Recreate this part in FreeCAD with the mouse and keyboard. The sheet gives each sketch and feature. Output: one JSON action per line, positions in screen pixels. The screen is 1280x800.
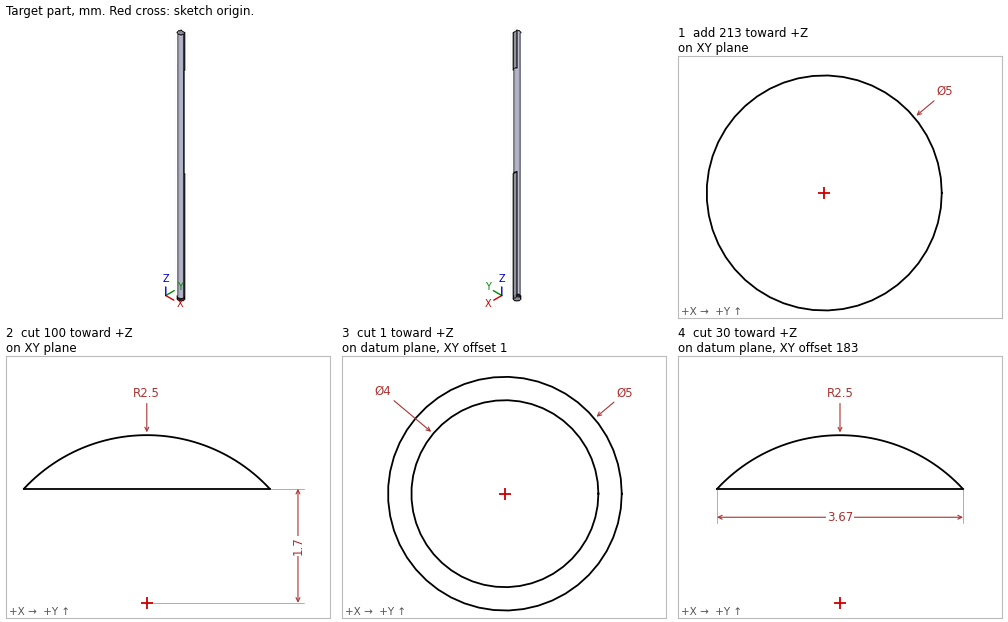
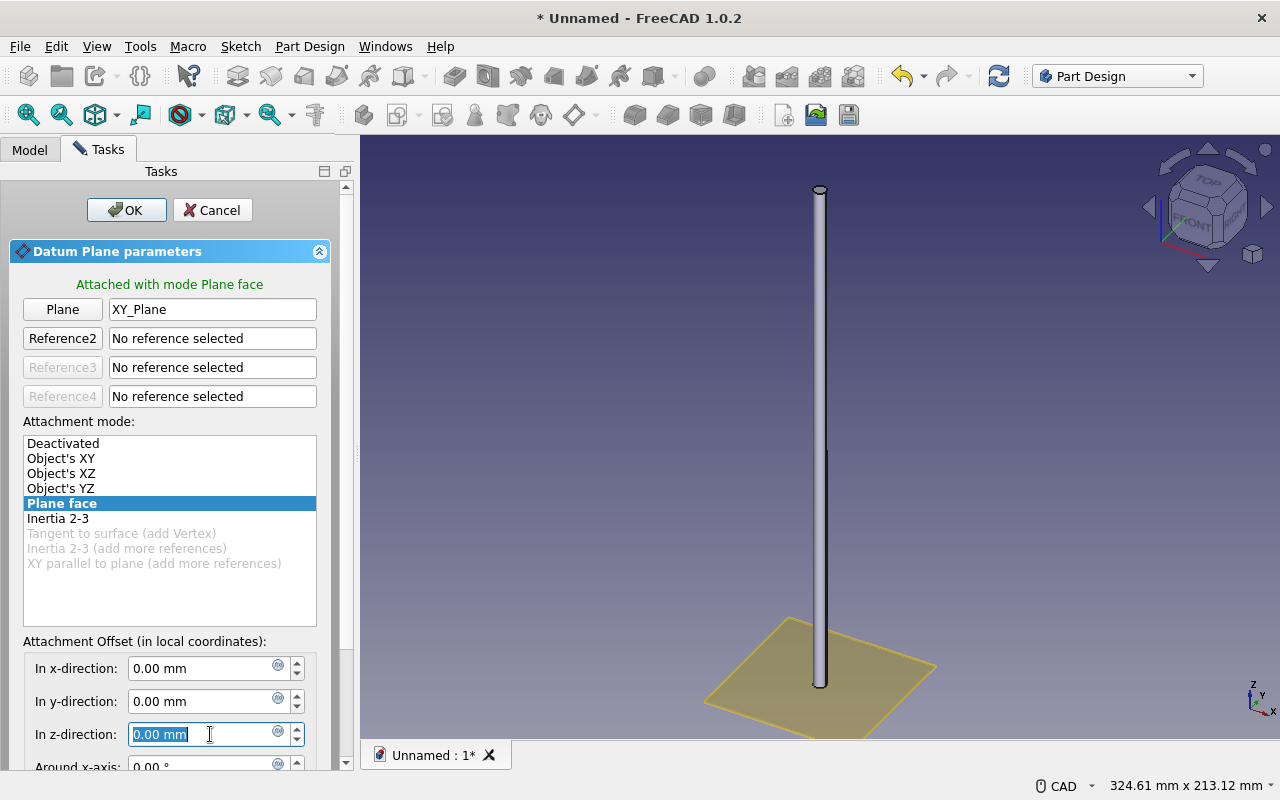
{"action": "type", "text": "1"}
{"action": "key", "text": "Tab"}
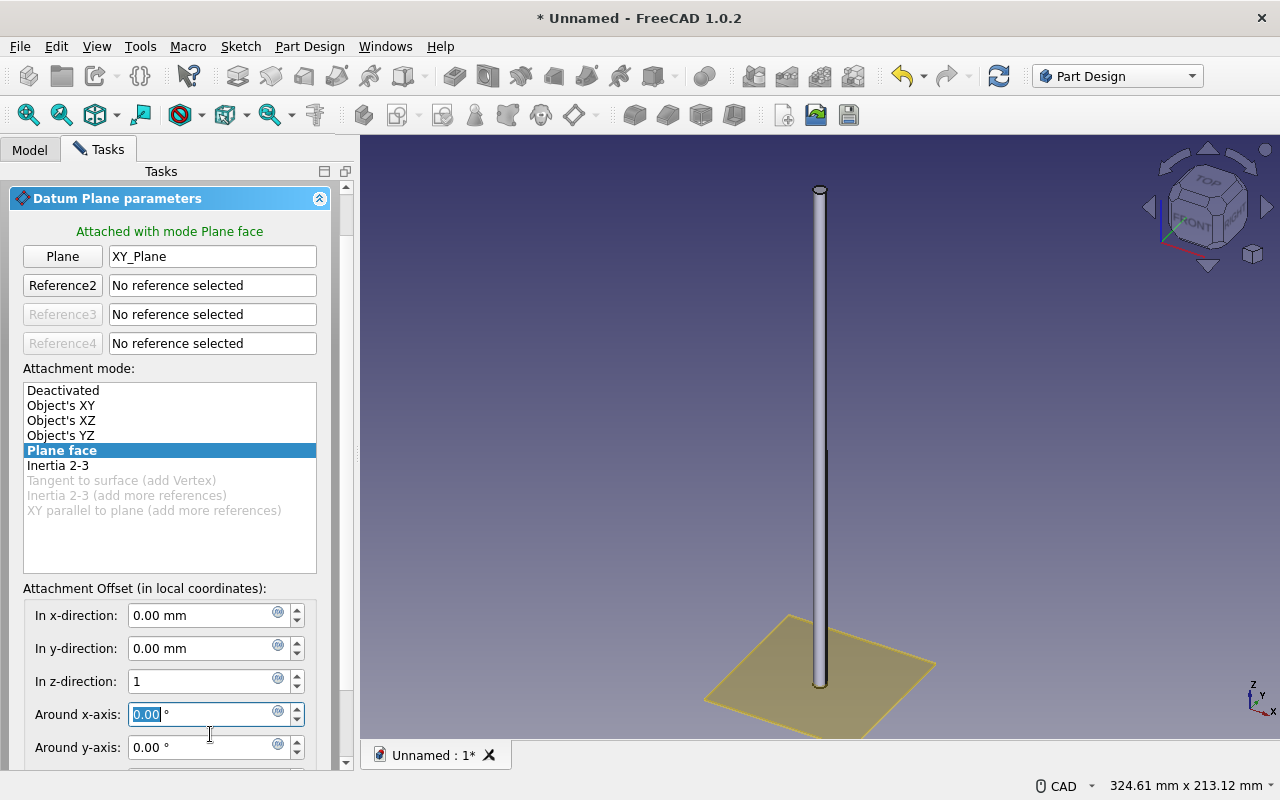
{"action": "scroll", "coordinate": [346, 476], "scroll_direction": "up", "scroll_amount": 2}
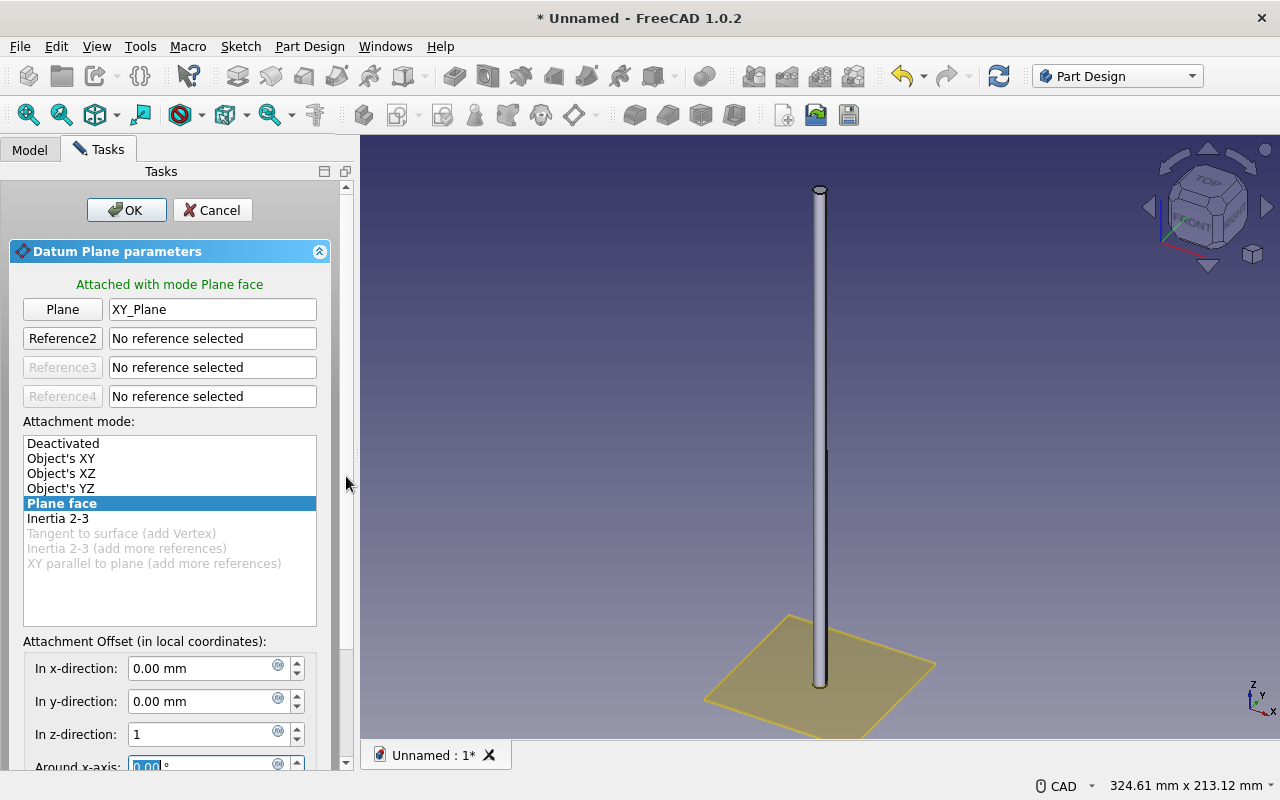
{"action": "left_click", "coordinate": [127, 210]}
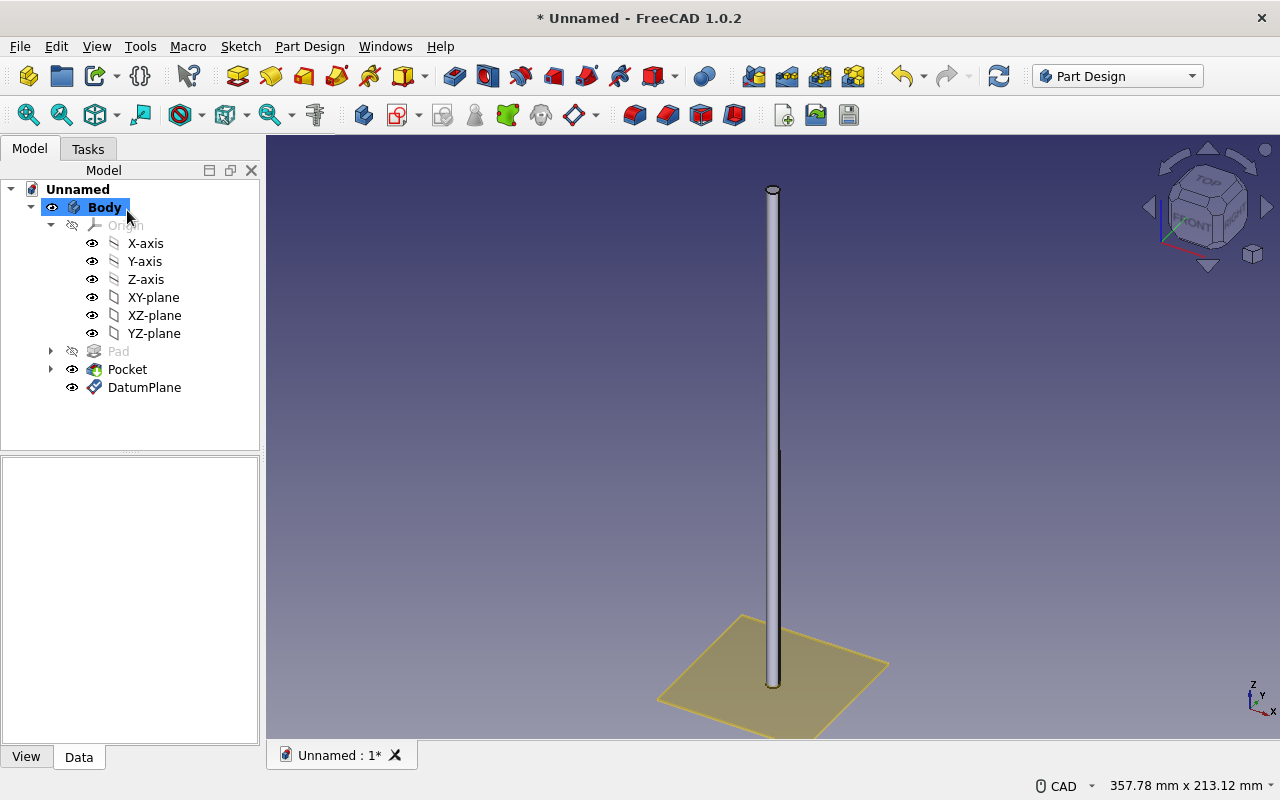
{"action": "left_click", "coordinate": [117, 387]}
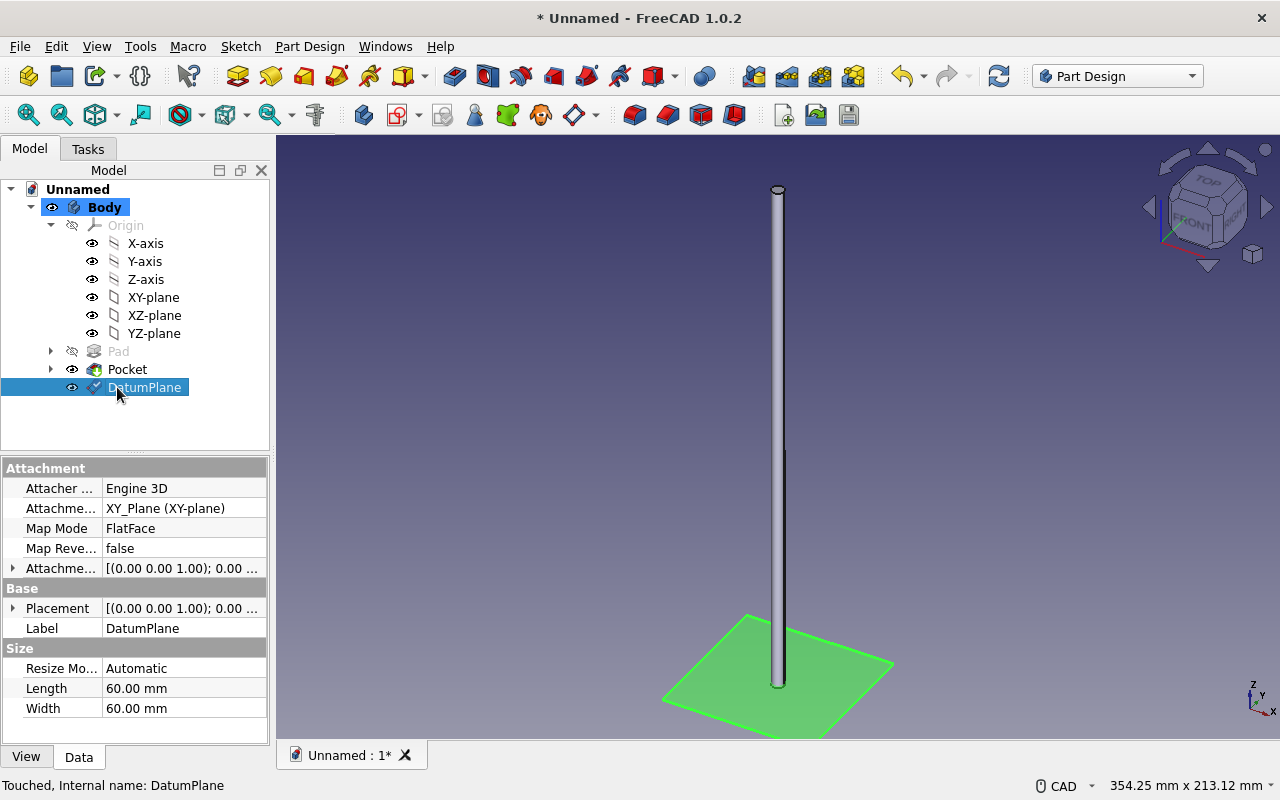
{"action": "left_click", "coordinate": [396, 116]}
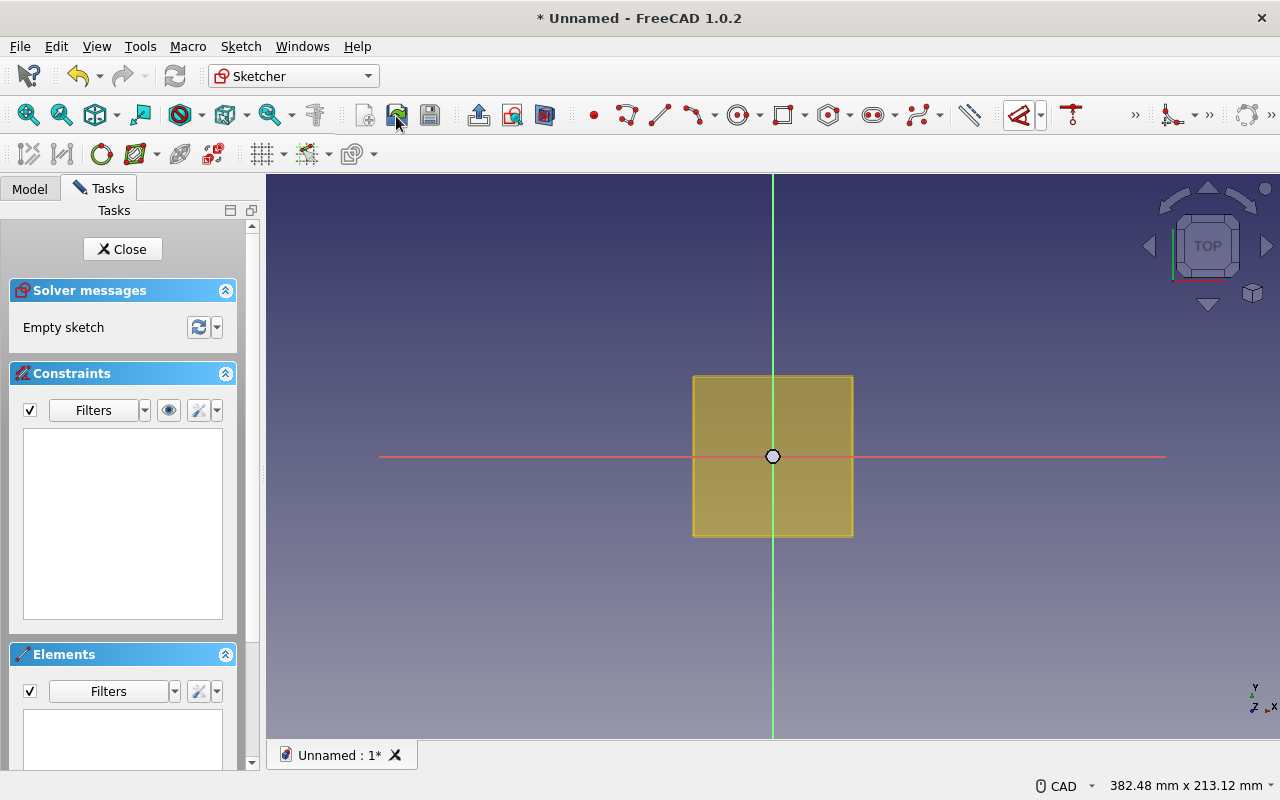
{"action": "key", "text": "q s"}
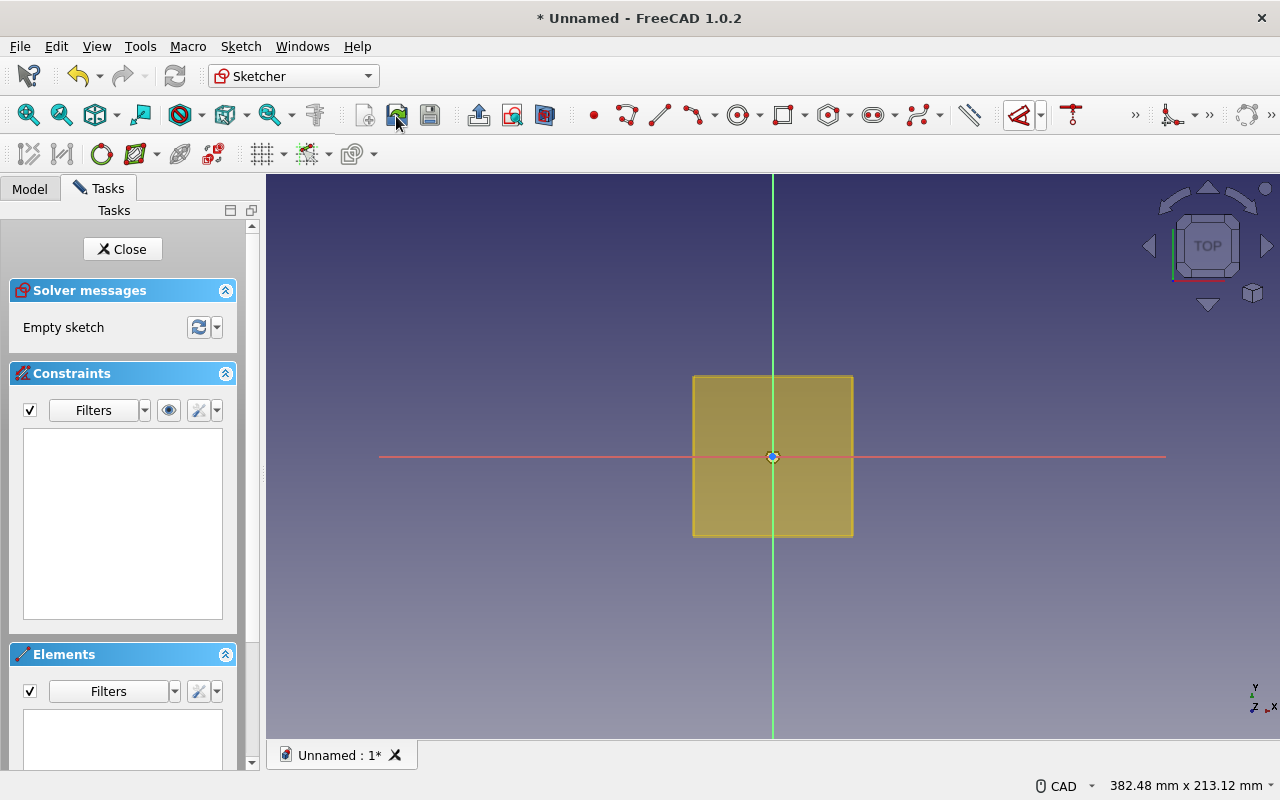
{"action": "scroll", "coordinate": [777, 456], "scroll_direction": "up", "scroll_amount": 15}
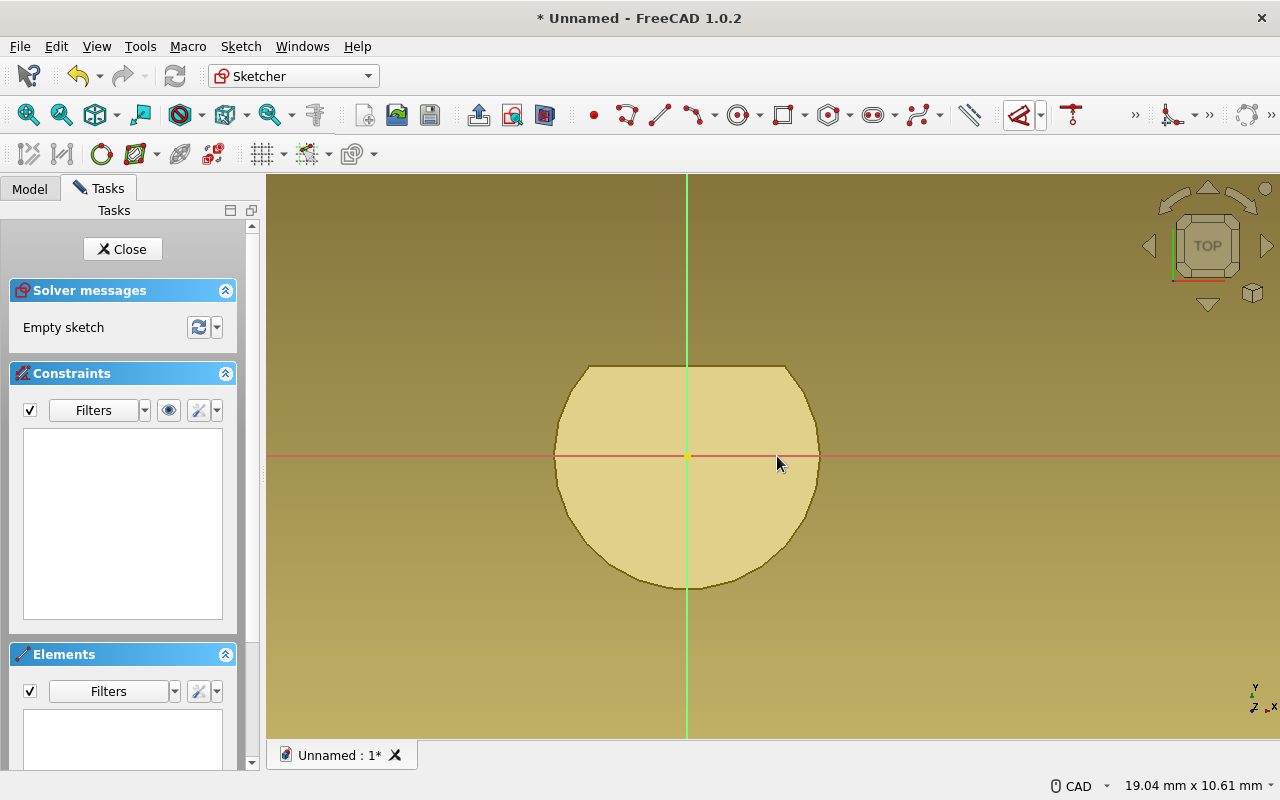
{"action": "left_click", "coordinate": [738, 116]}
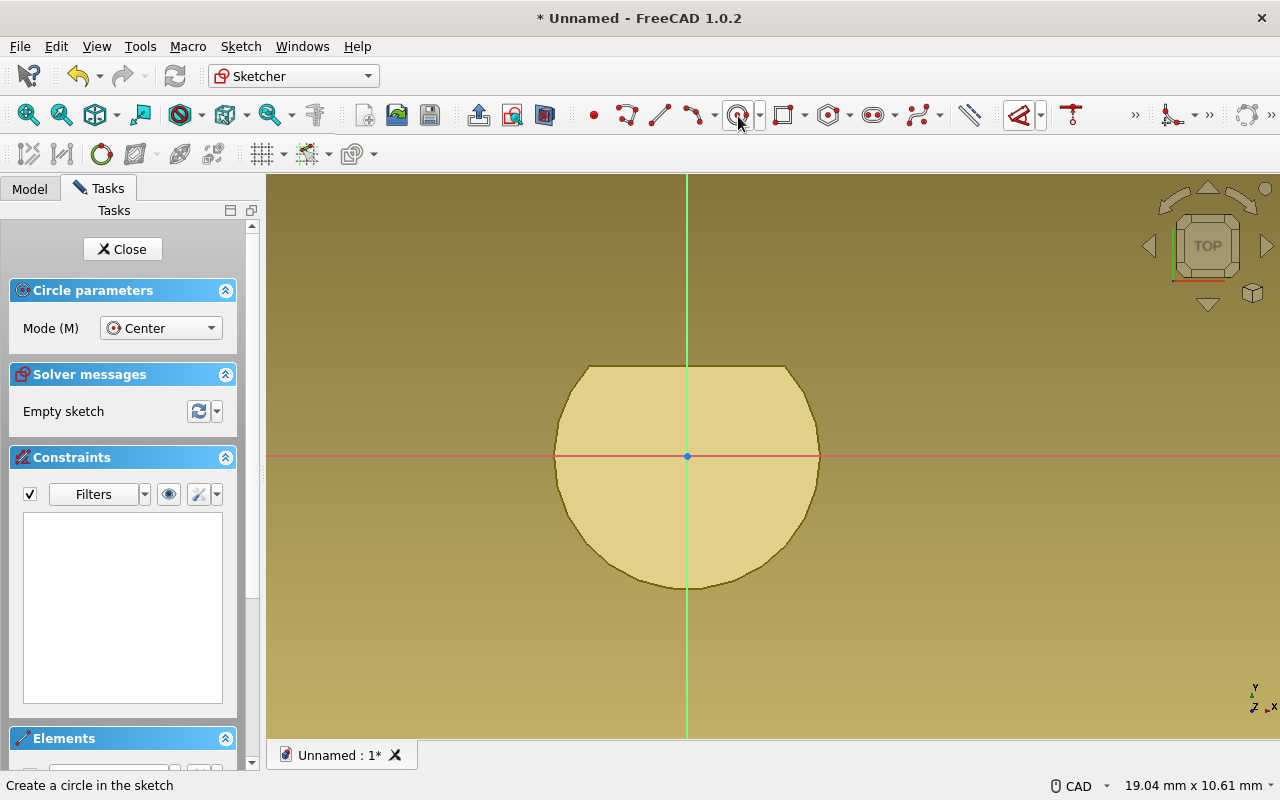
{"action": "left_click", "coordinate": [687, 456]}
{"action": "mouse_move", "coordinate": [781, 362]}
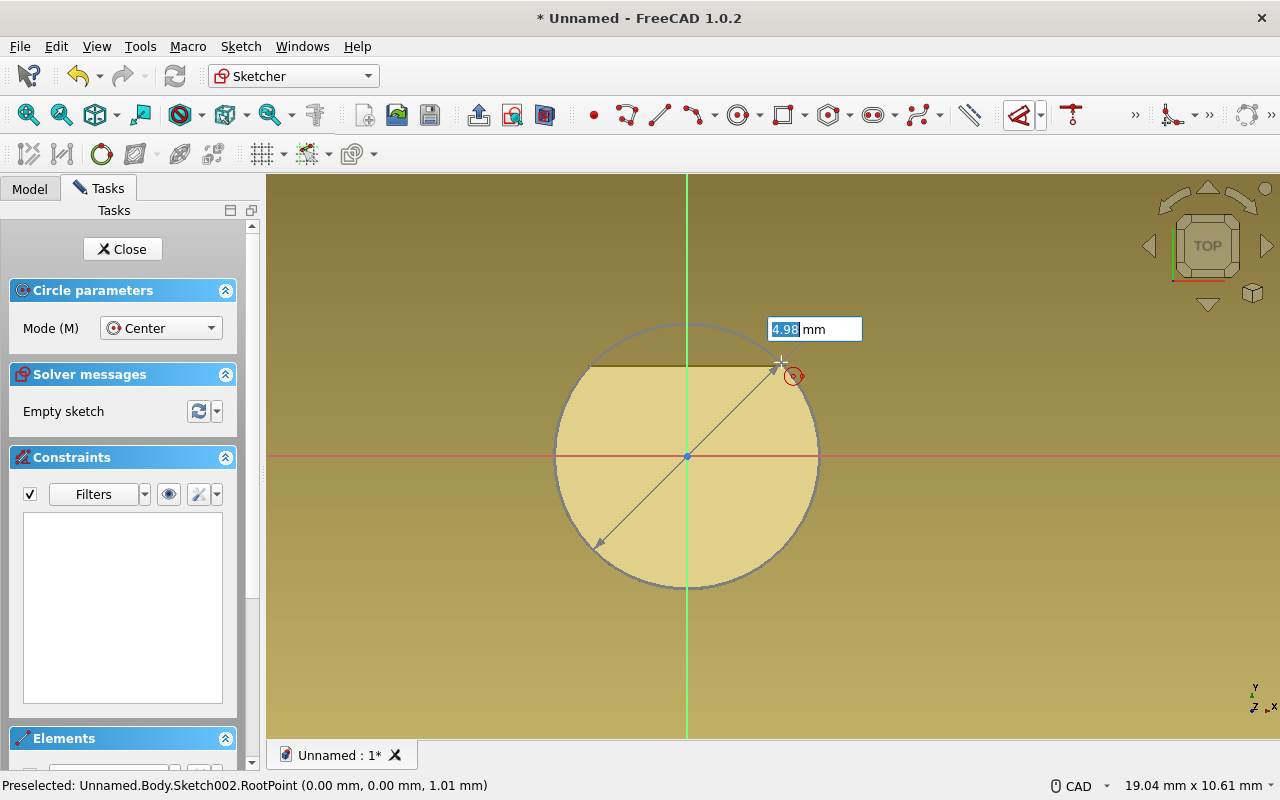
{"action": "type", "text": "5"}
{"action": "key", "text": "Return"}